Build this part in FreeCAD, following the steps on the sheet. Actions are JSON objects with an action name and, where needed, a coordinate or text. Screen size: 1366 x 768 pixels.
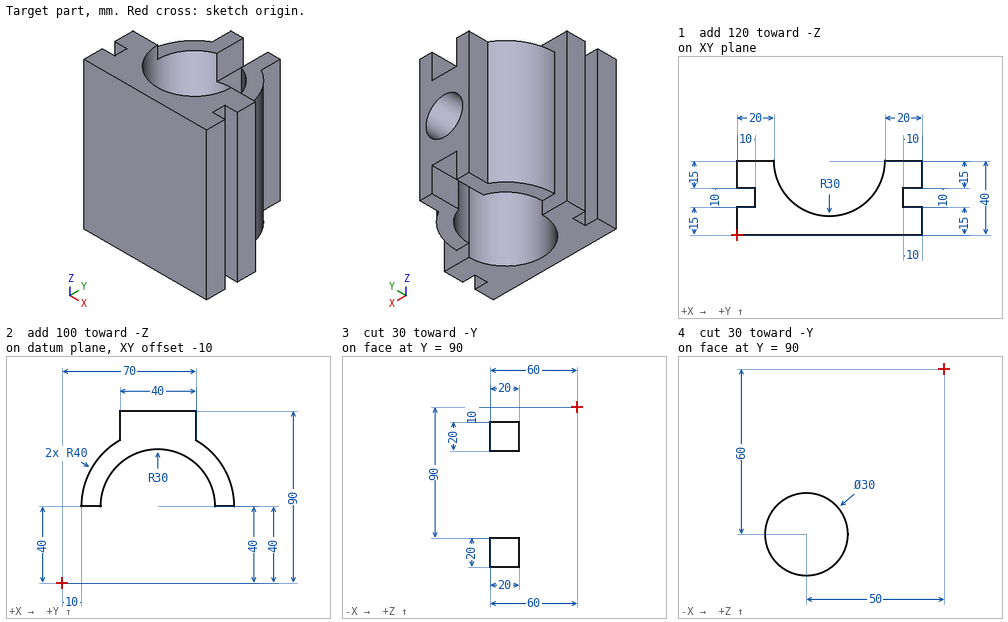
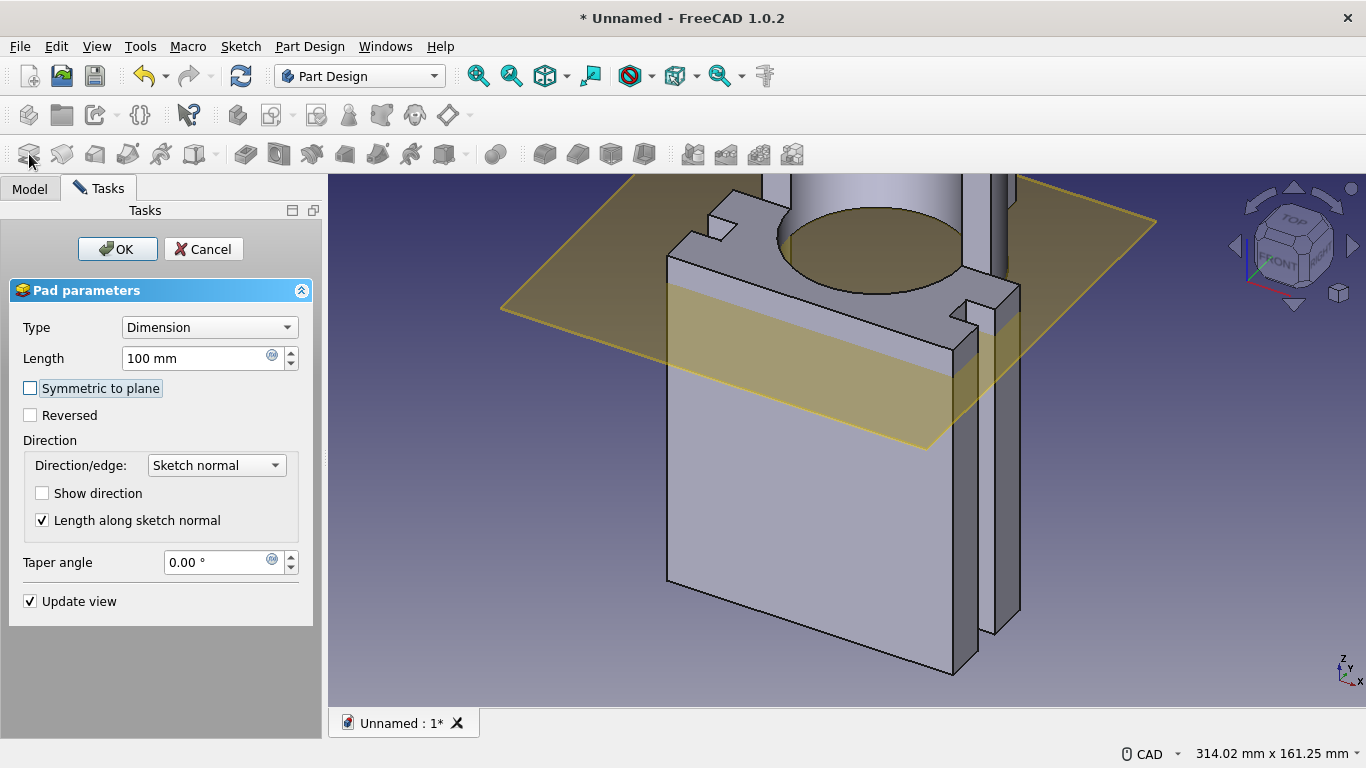
{"action": "left_click", "coordinate": [31, 415]}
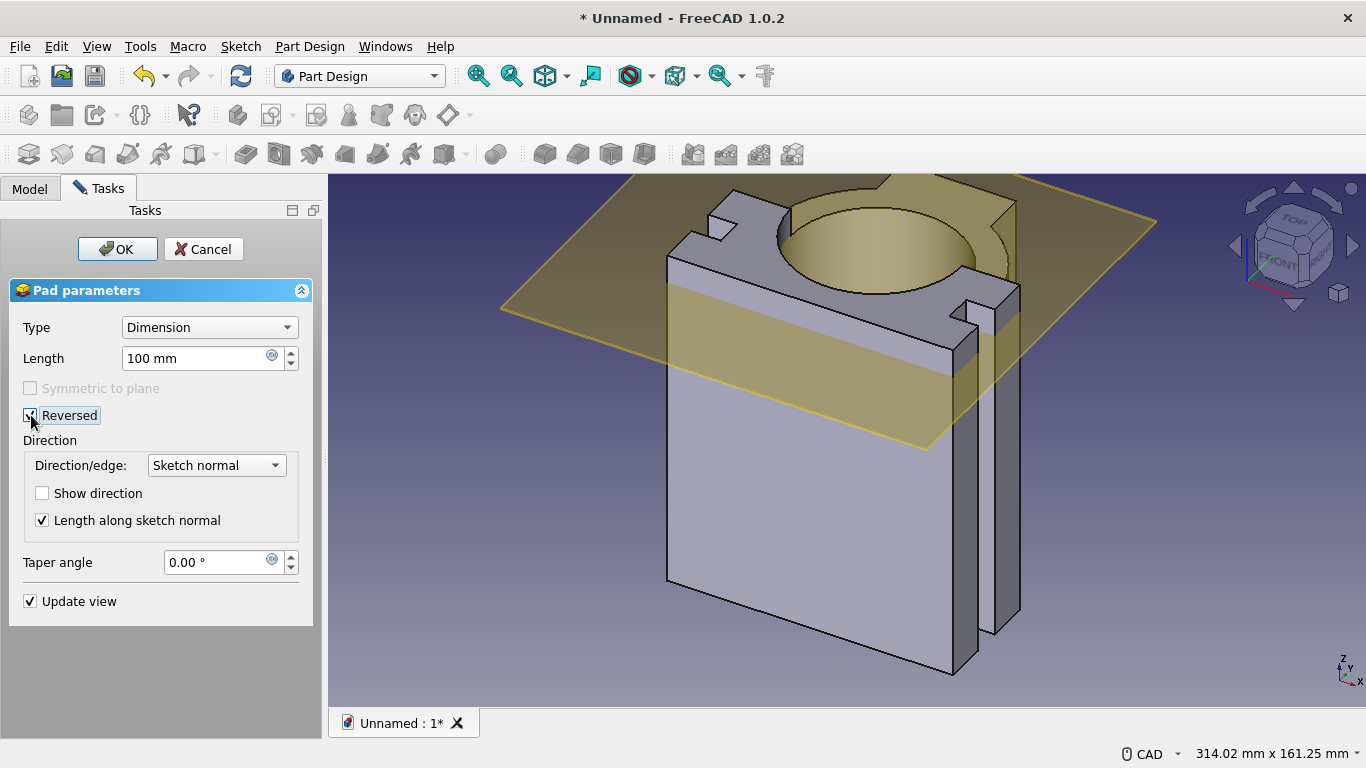
{"action": "left_click", "coordinate": [118, 249]}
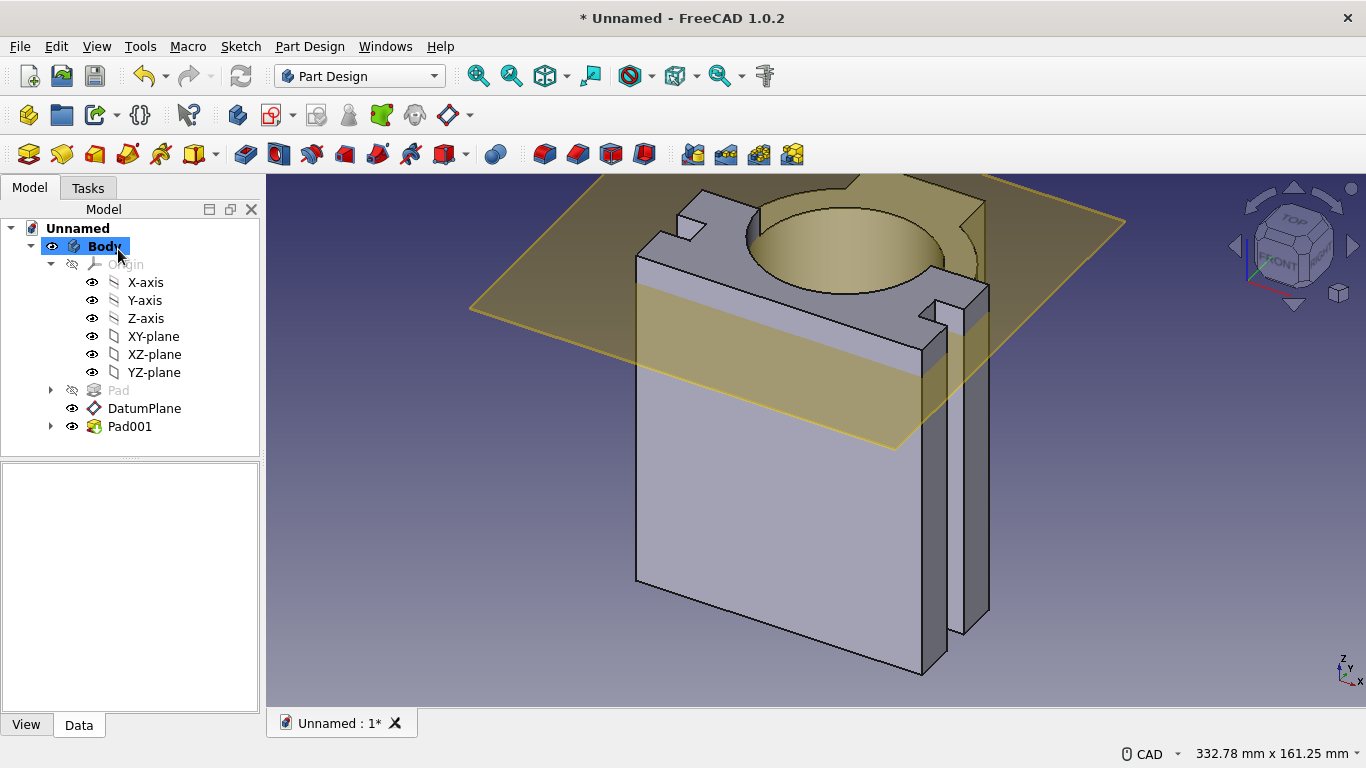
{"action": "left_click", "coordinate": [117, 408]}
{"action": "key", "text": "space"}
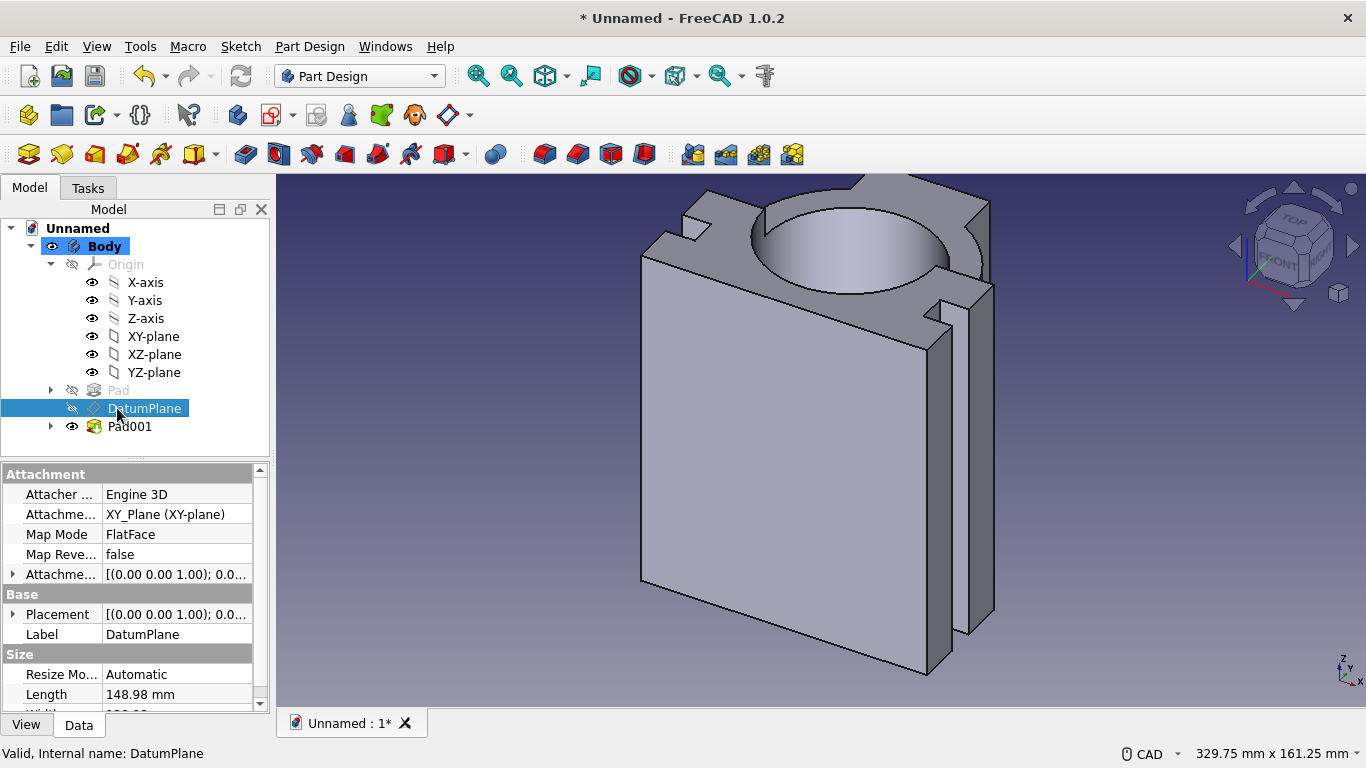
{"action": "left_click", "coordinate": [479, 76]}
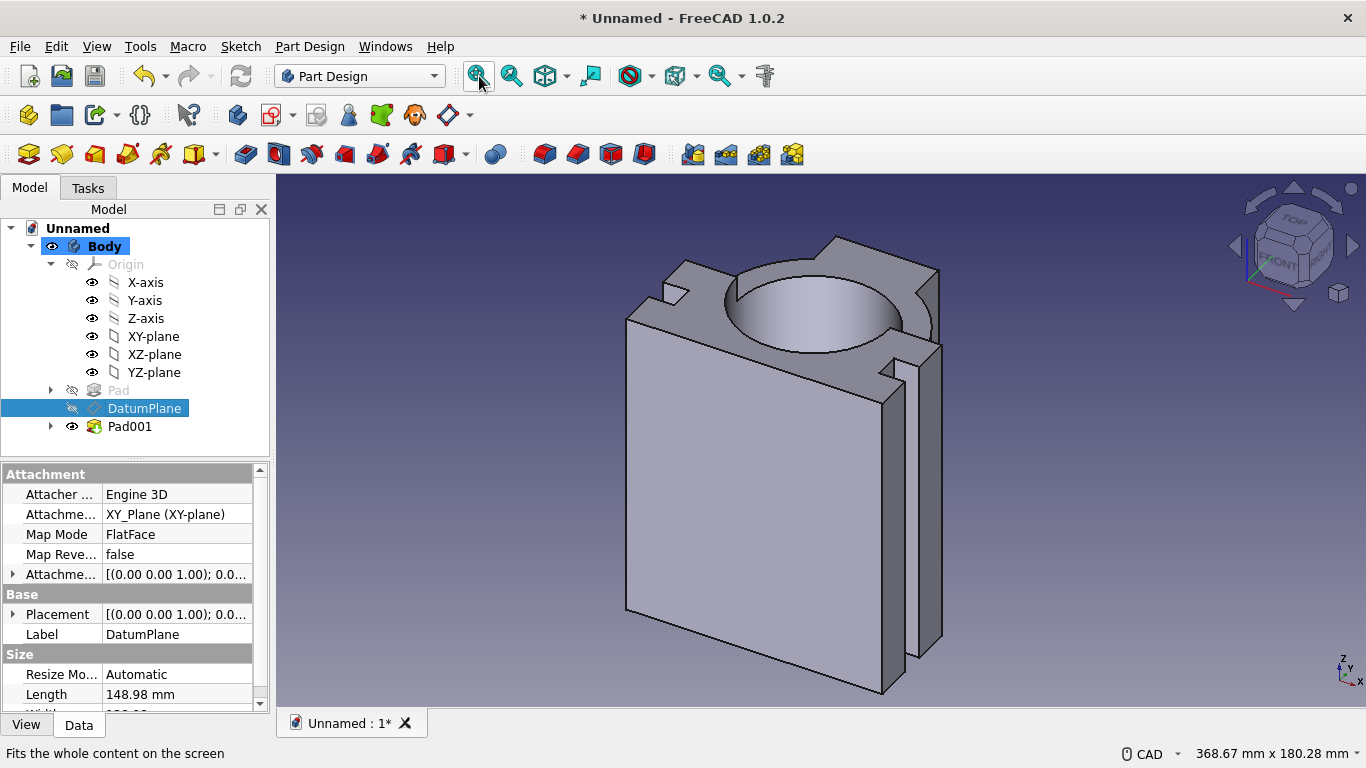
{"action": "key", "text": "4"}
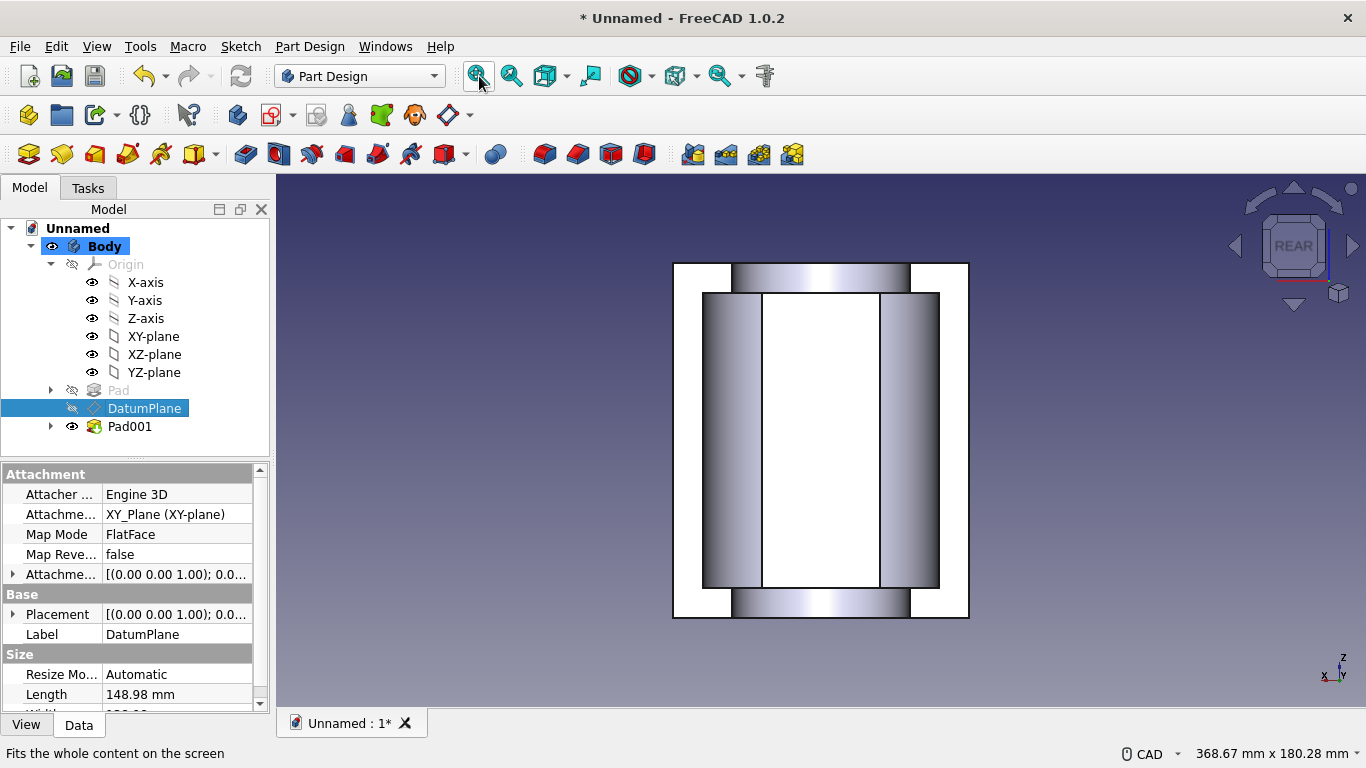
{"action": "left_click", "coordinate": [821, 355]}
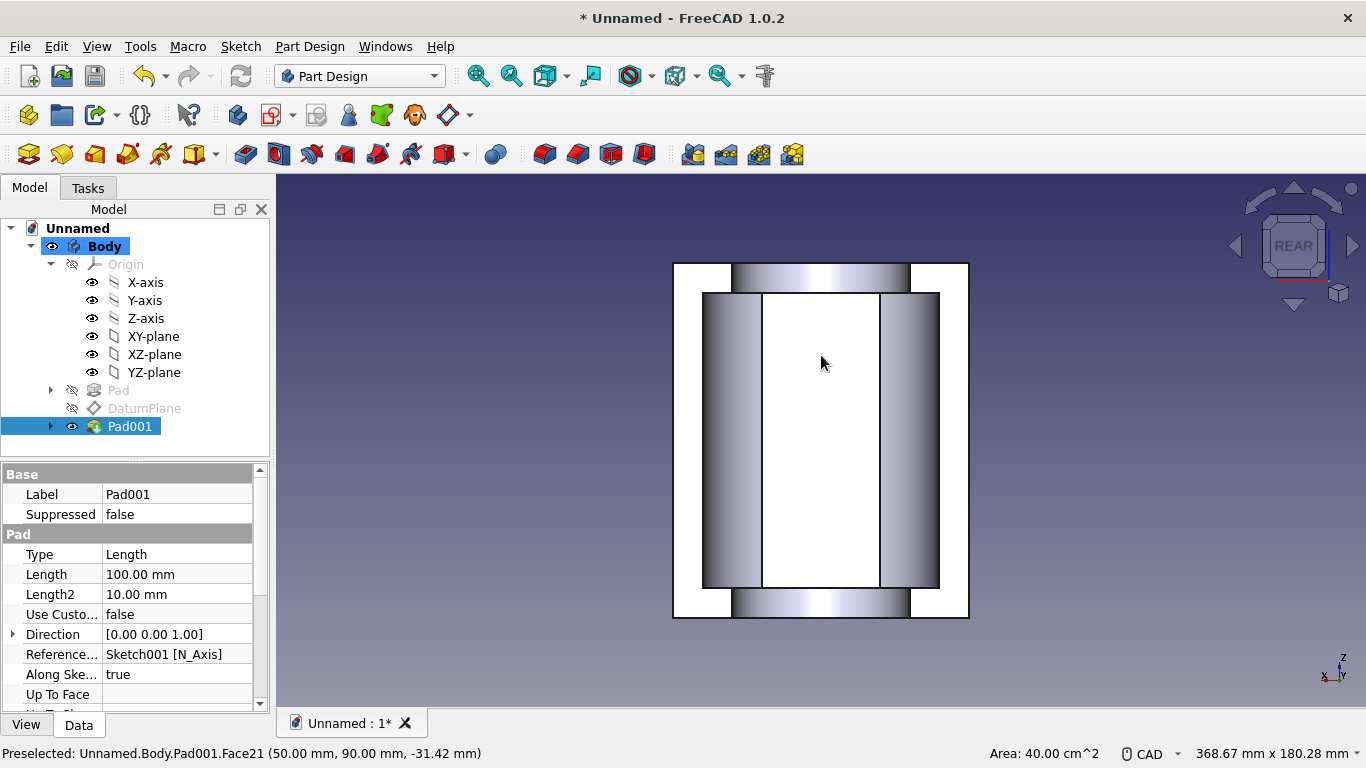
{"action": "left_click", "coordinate": [270, 116]}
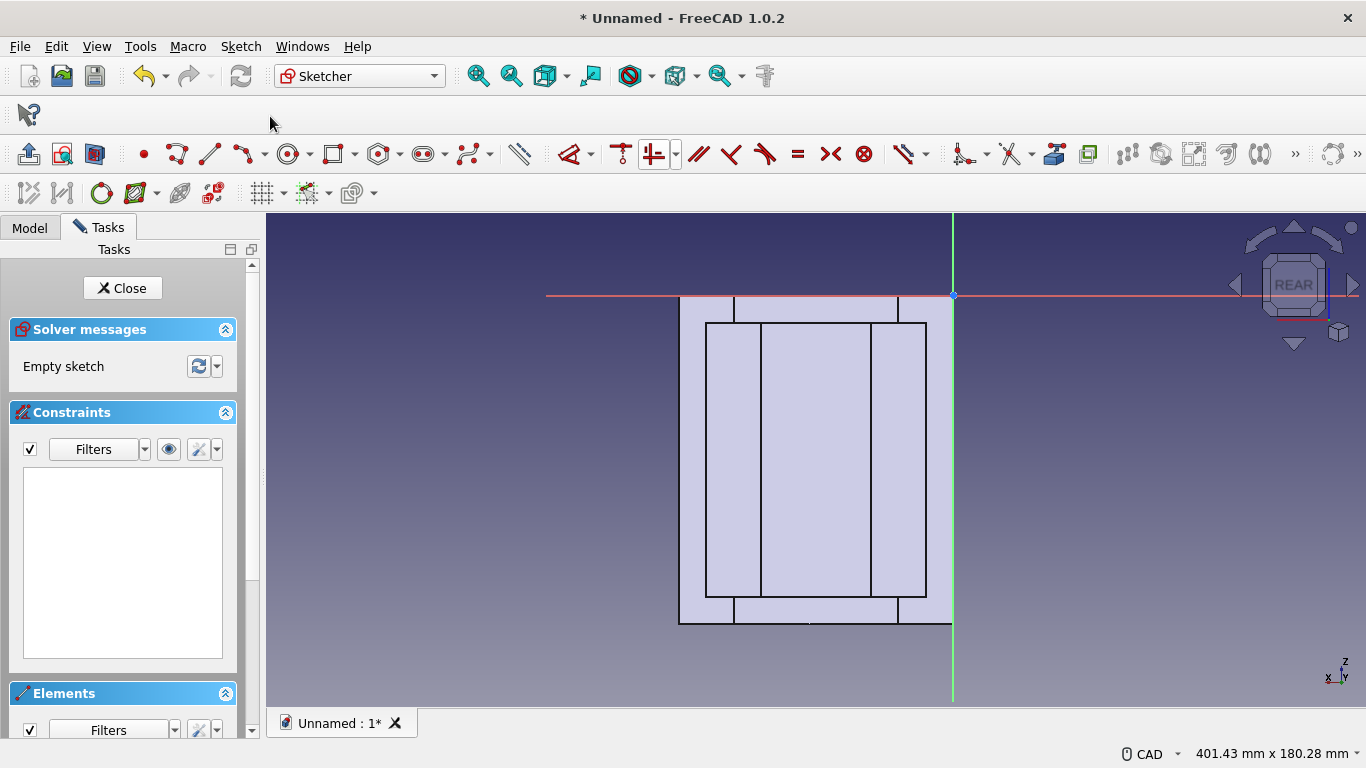
{"action": "left_click", "coordinate": [332, 154]}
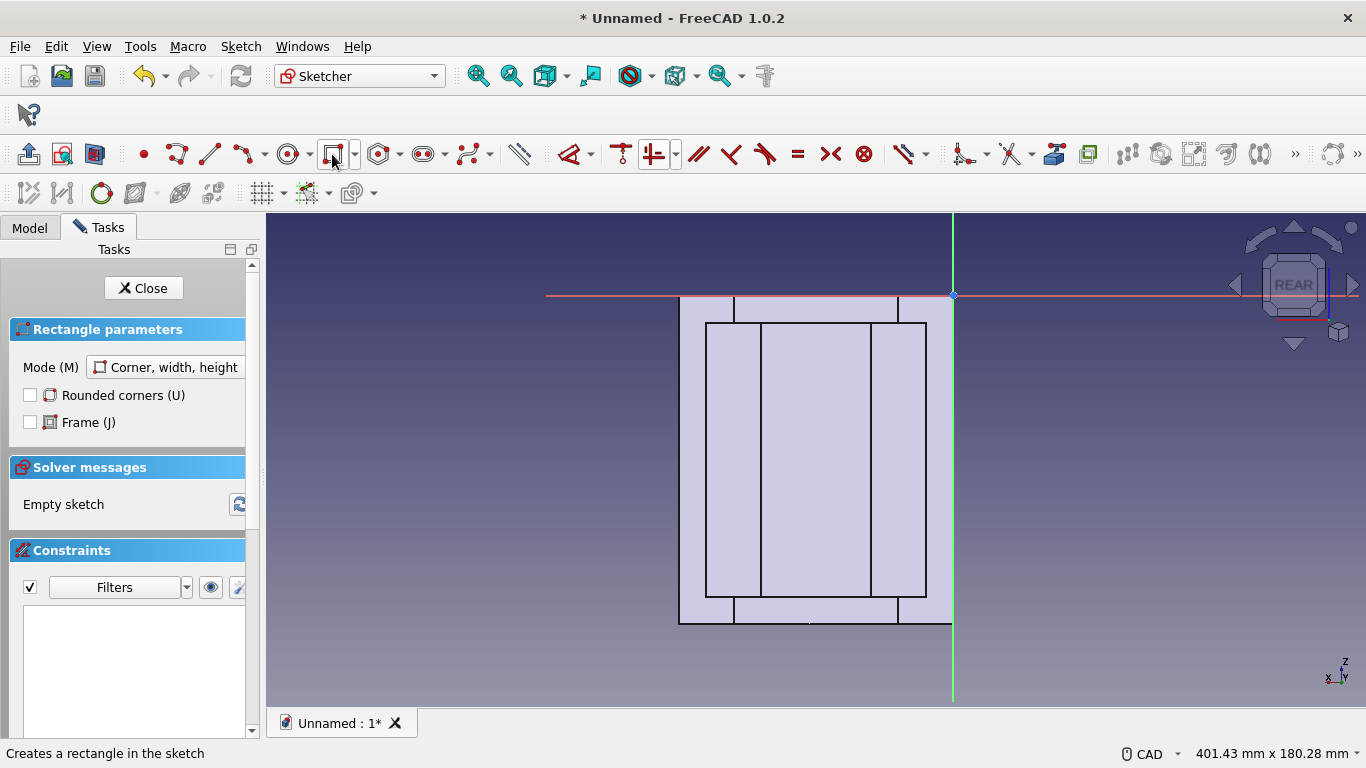
{"action": "left_click", "coordinate": [789, 323]}
{"action": "left_click", "coordinate": [843, 378]}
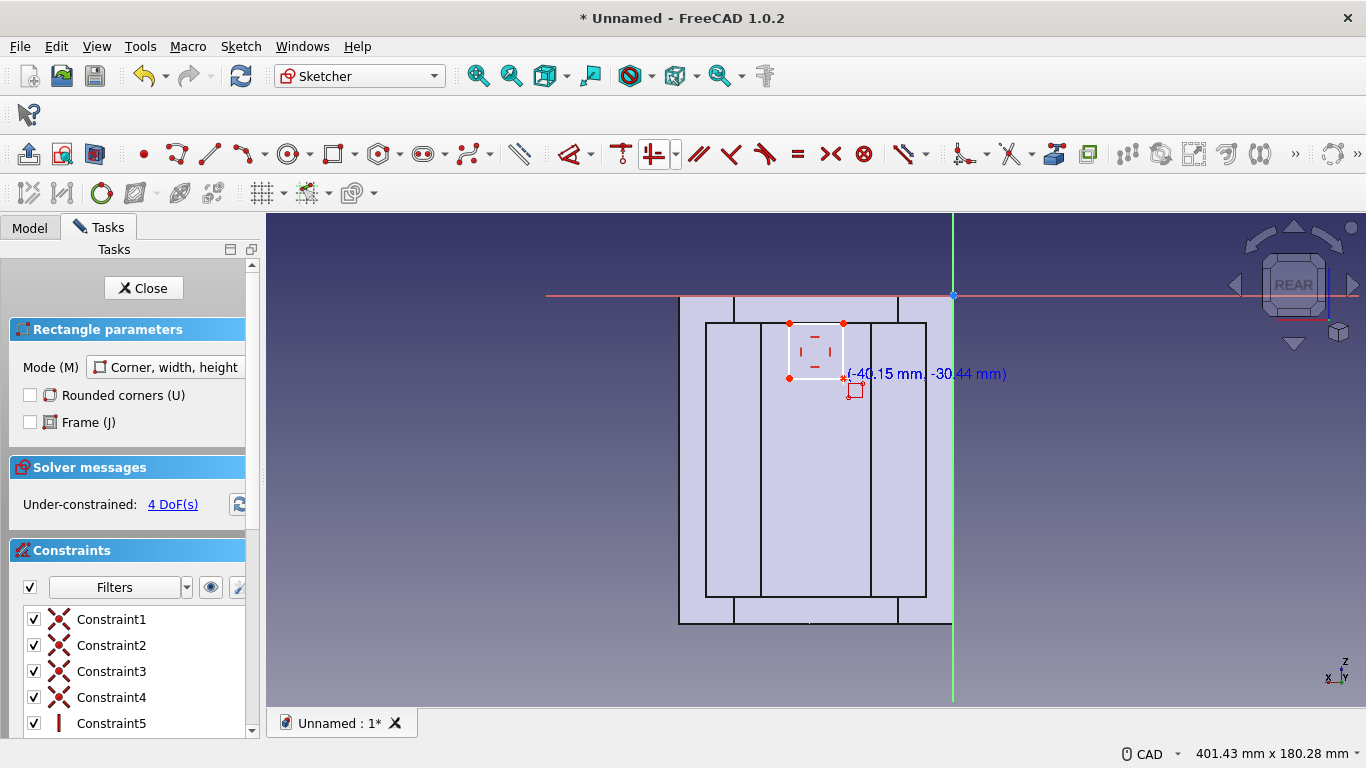
{"action": "left_click", "coordinate": [789, 542]}
{"action": "left_click", "coordinate": [843, 597]}
{"action": "key", "text": "Escape"}